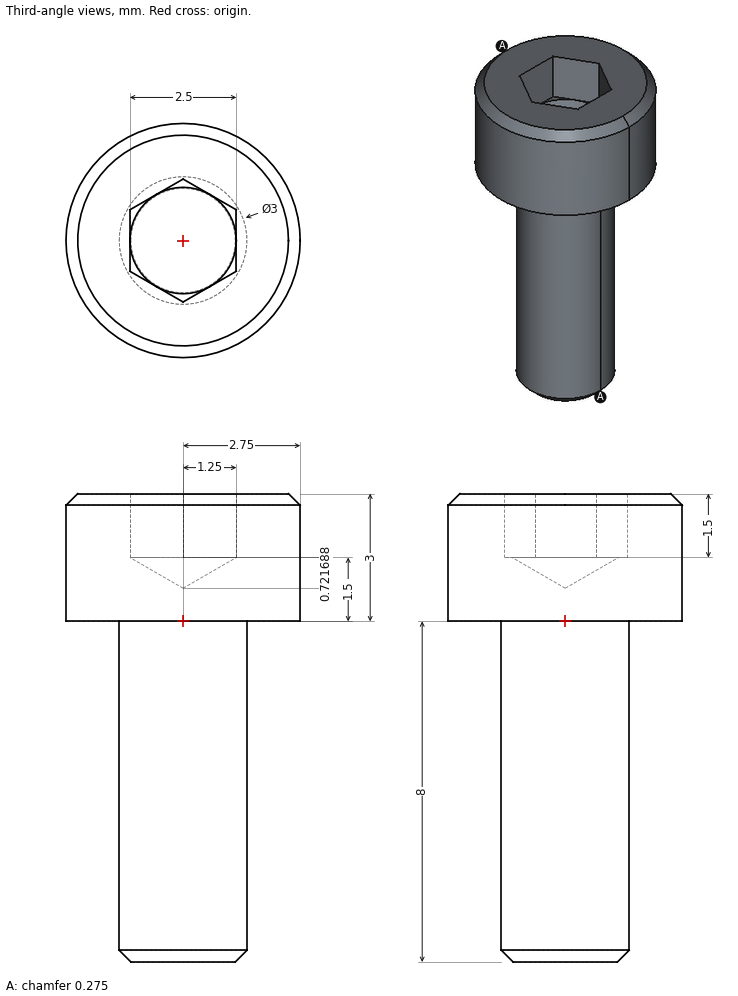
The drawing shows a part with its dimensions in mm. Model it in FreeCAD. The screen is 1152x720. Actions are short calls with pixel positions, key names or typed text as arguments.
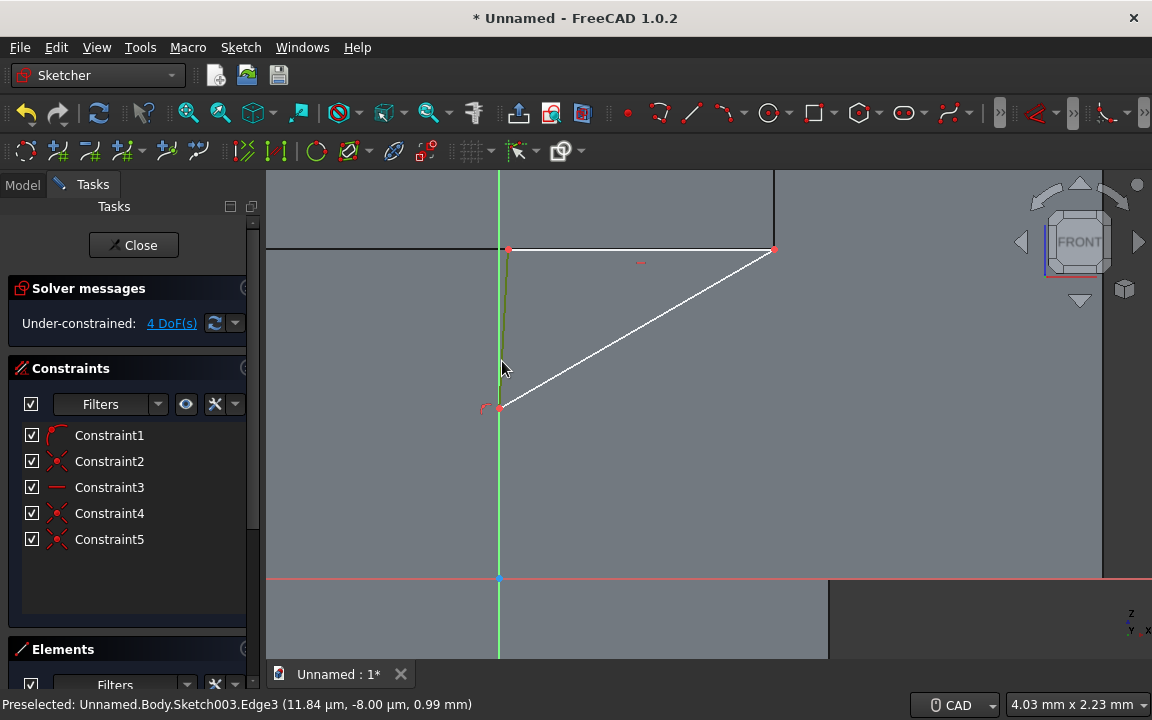
key(v)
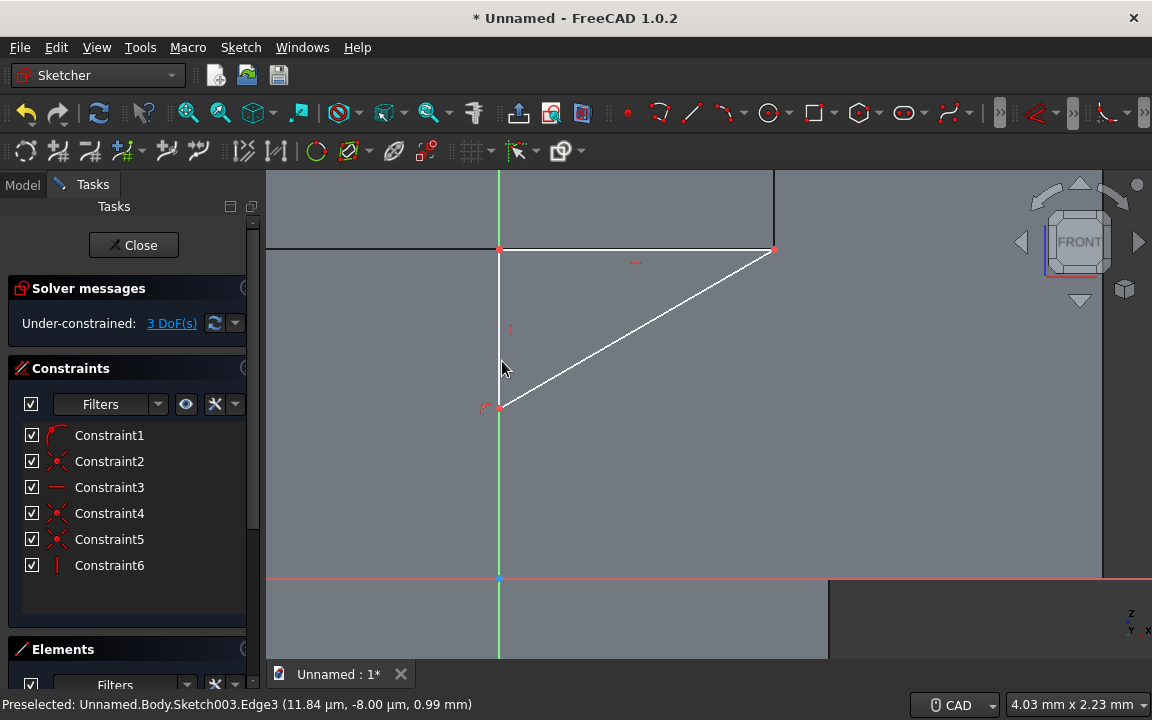
click(692, 250)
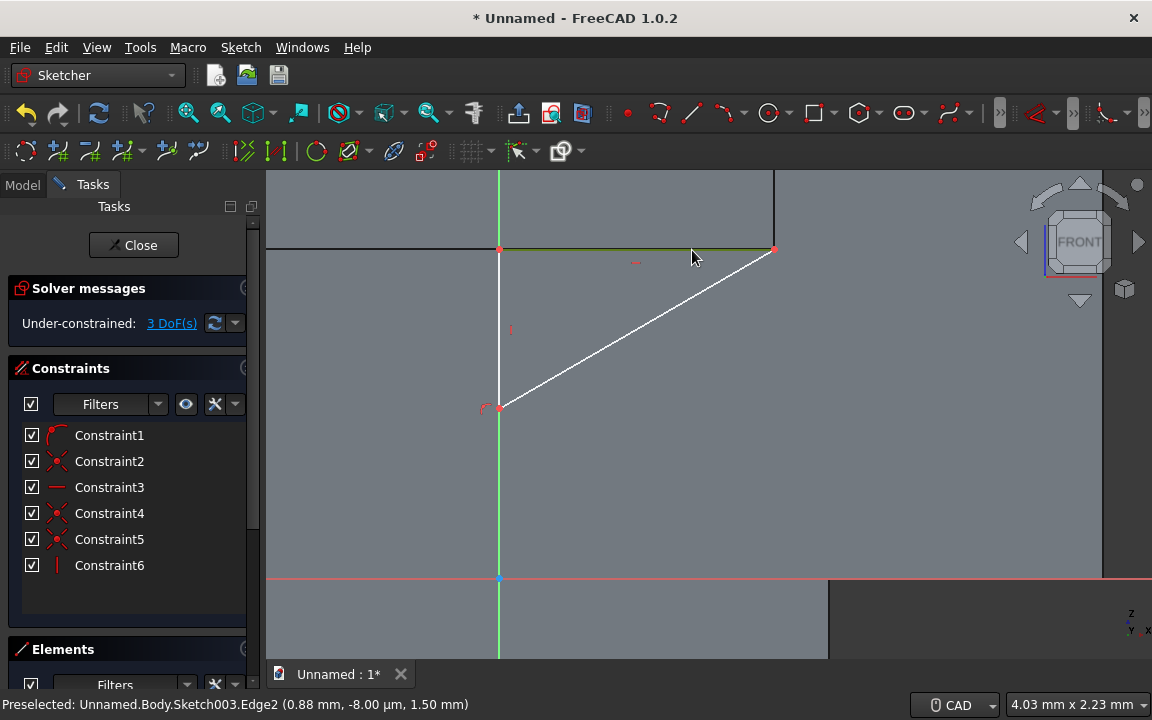
click(1058, 114)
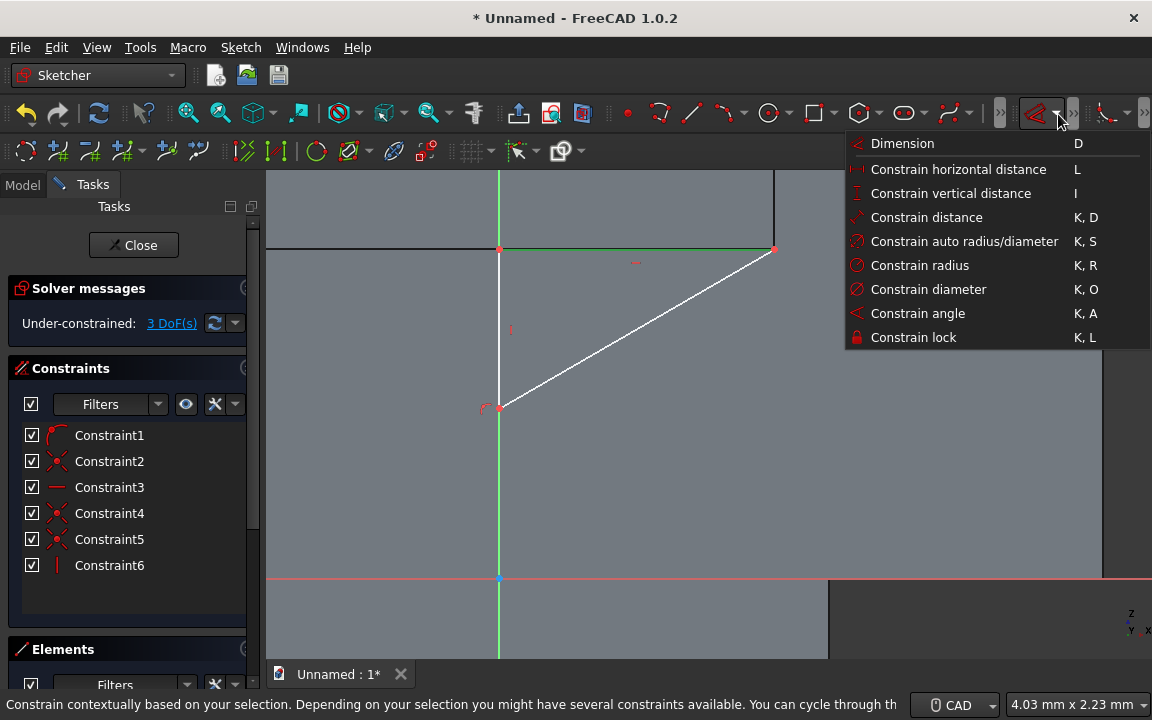
click(998, 169)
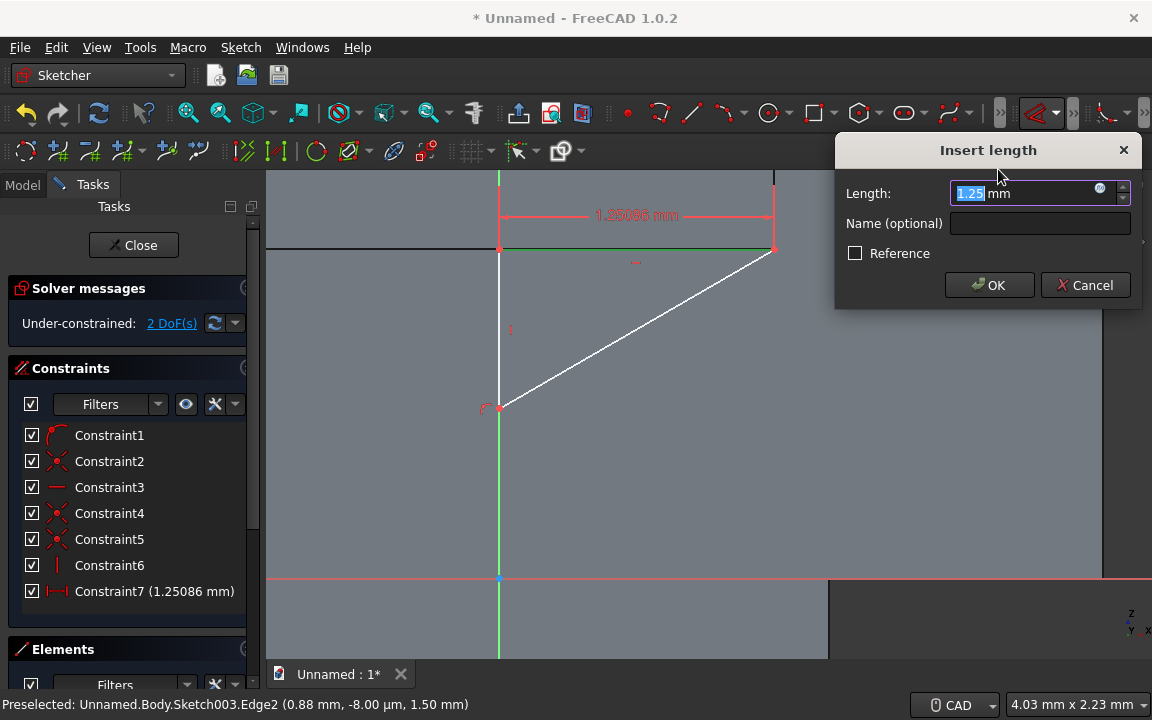
text(1.25)
key(Return)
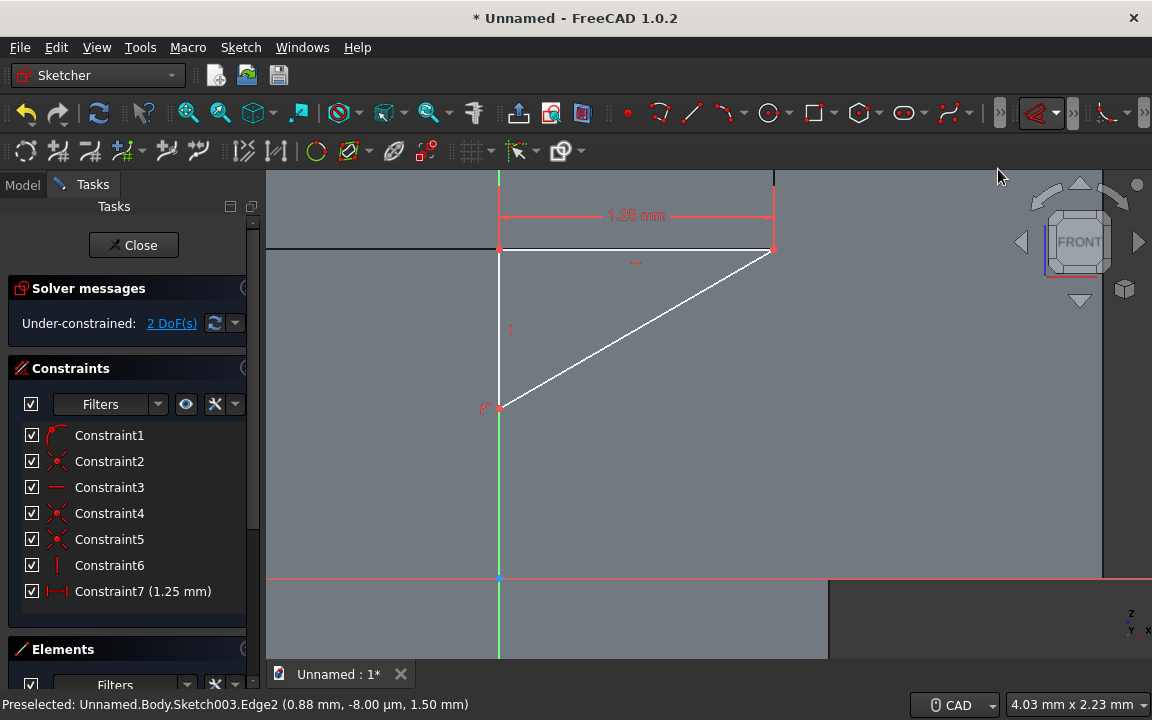
click(774, 250)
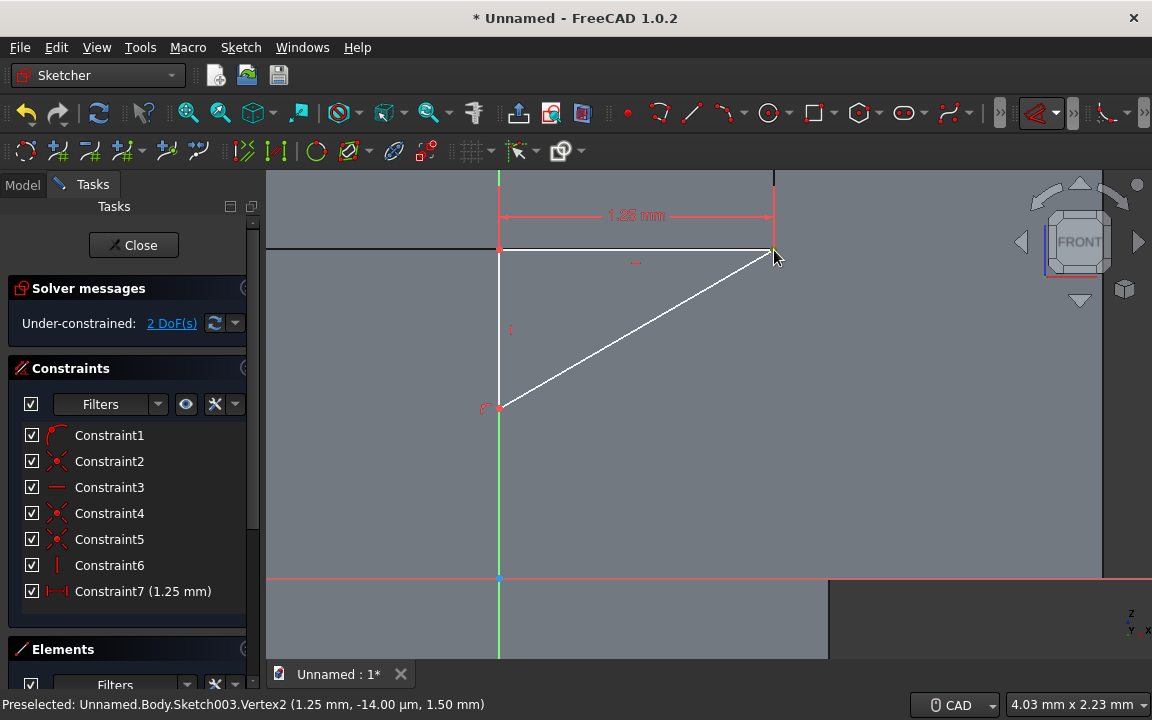
key(i)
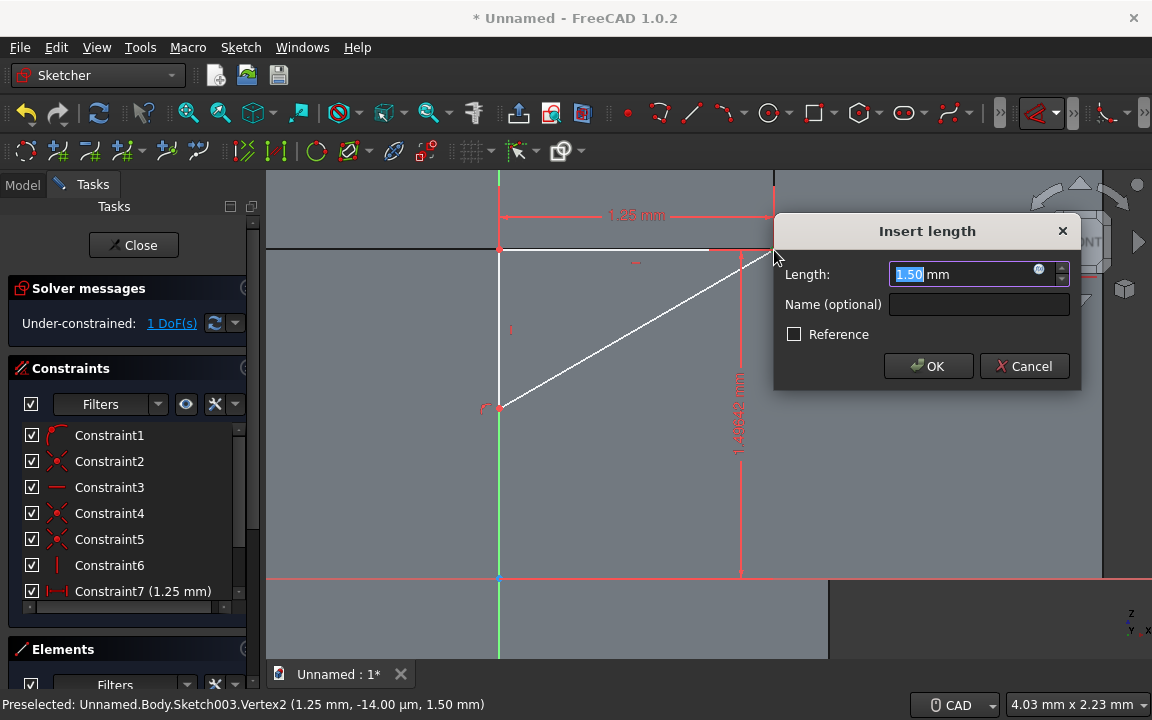
text(1.5)
key(Return)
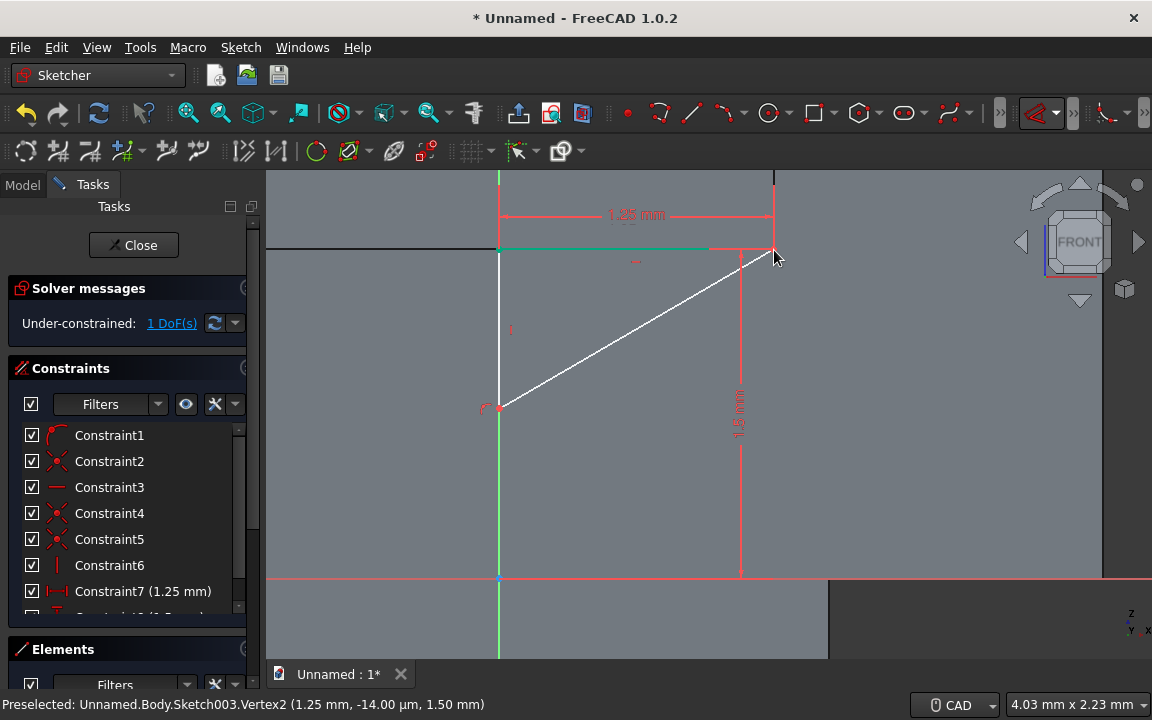
click(499, 297)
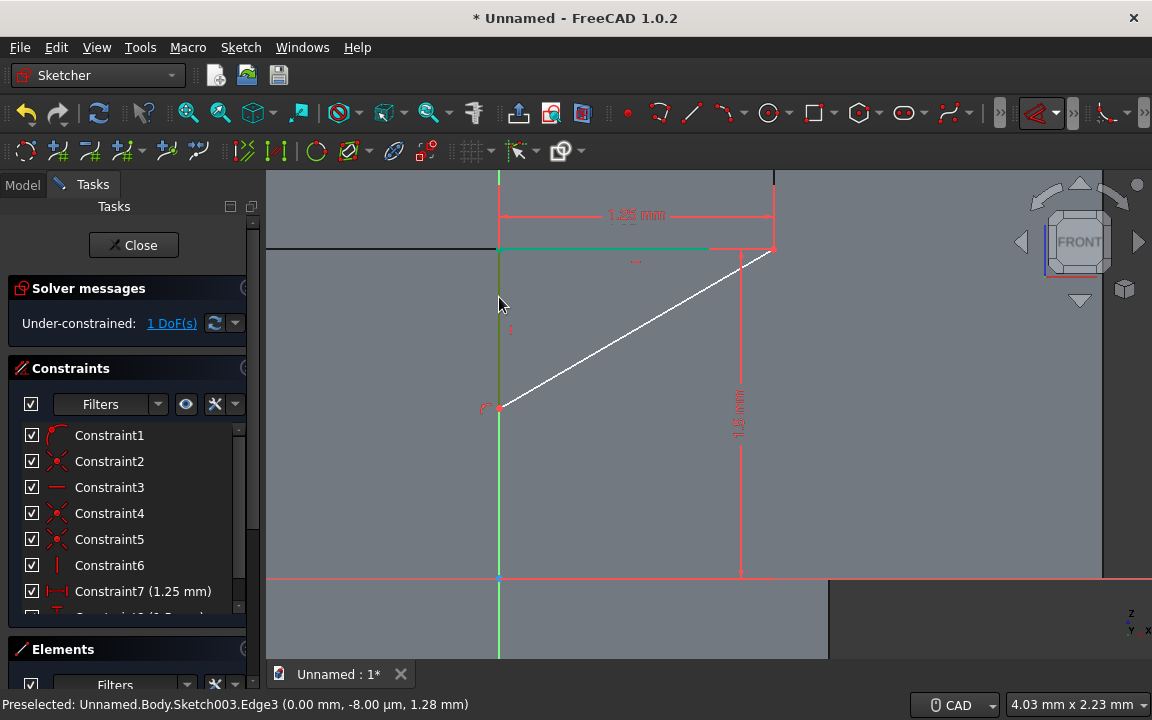
key(i)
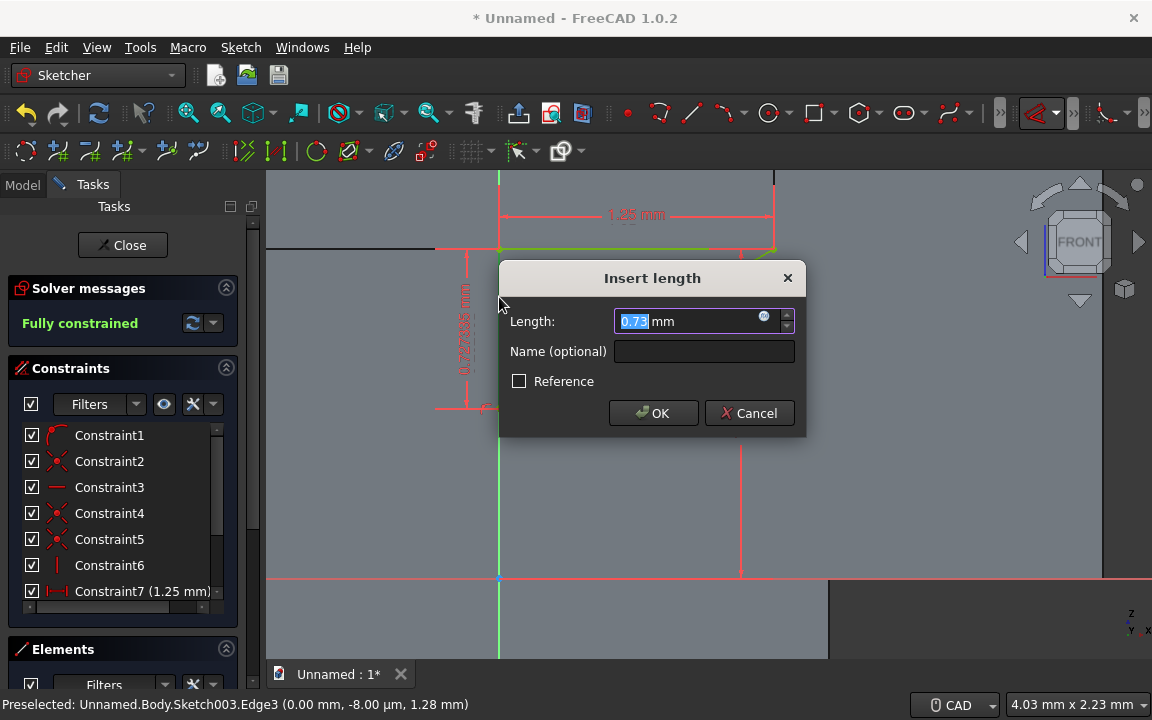
text(0.721688)
key(Return)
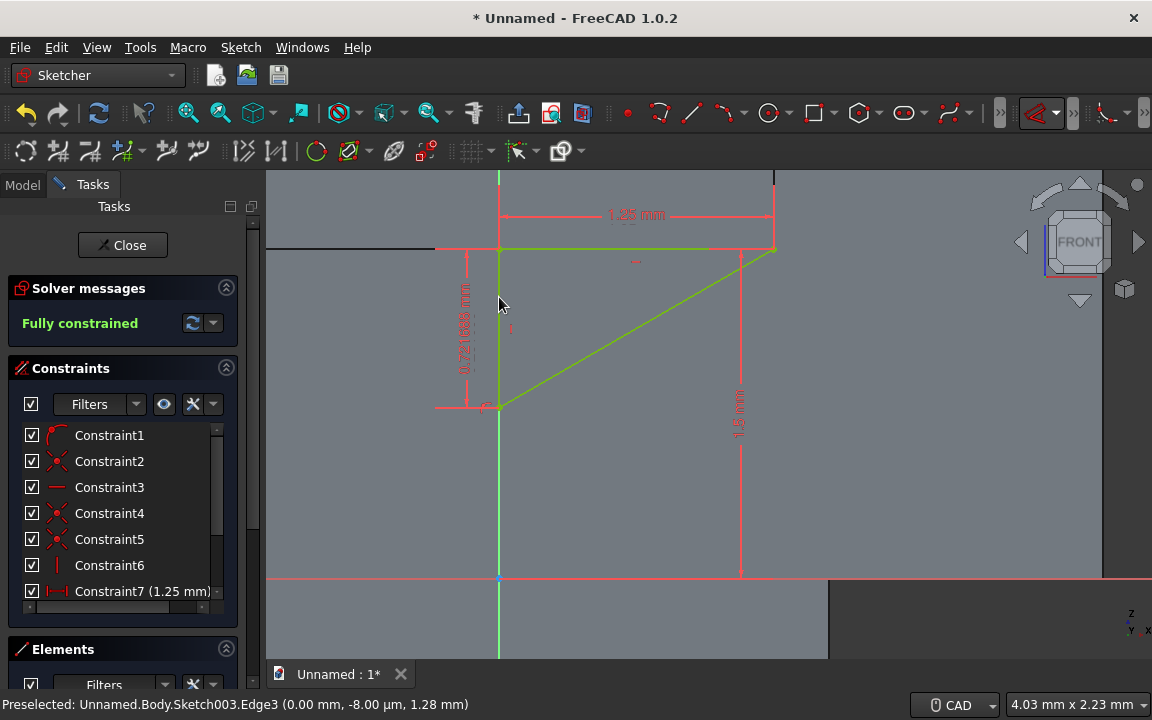
click(123, 245)